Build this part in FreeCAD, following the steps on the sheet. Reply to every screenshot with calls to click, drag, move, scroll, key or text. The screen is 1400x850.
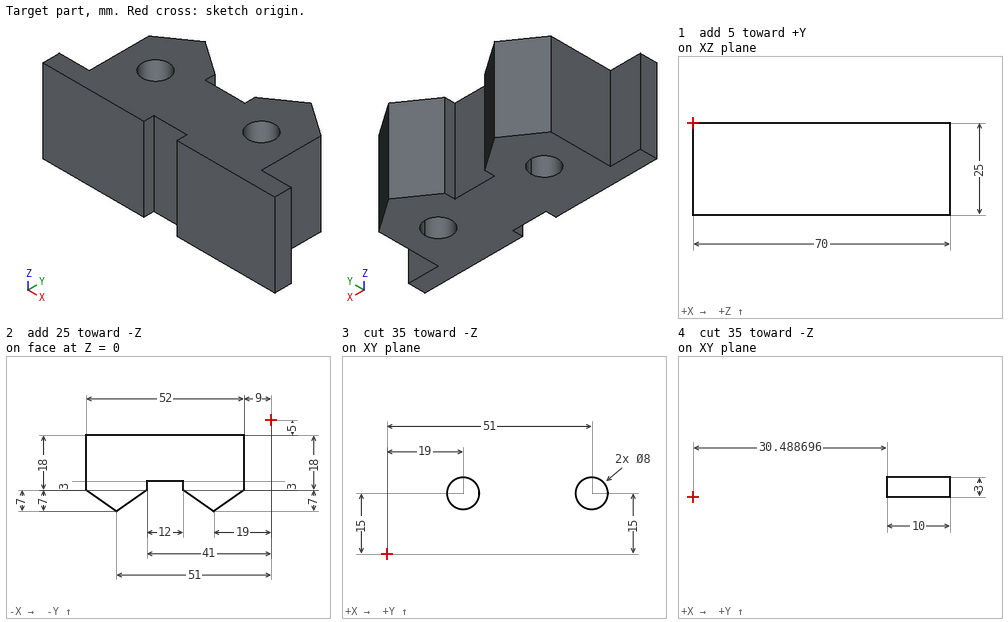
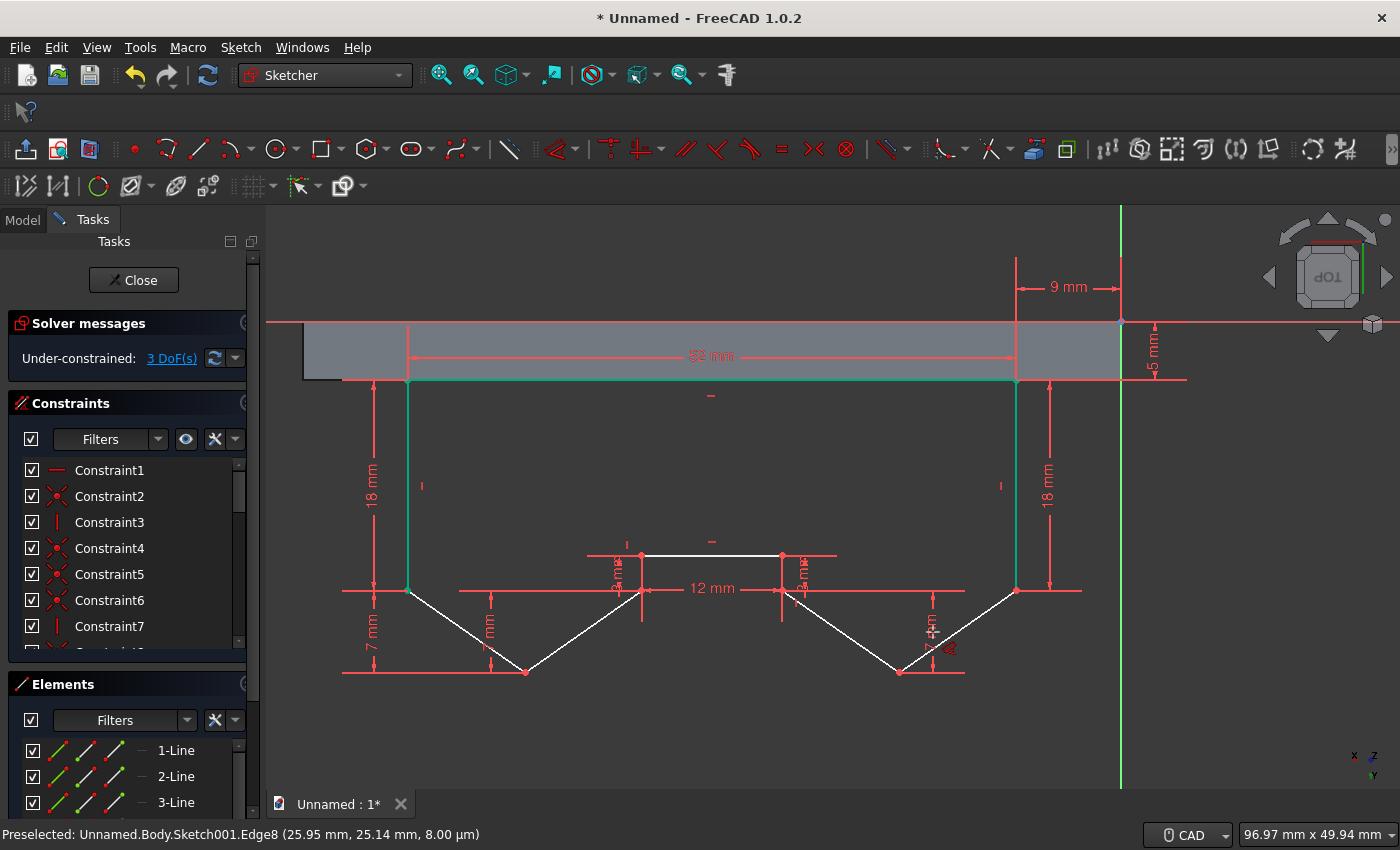
click(525, 673)
click(823, 707)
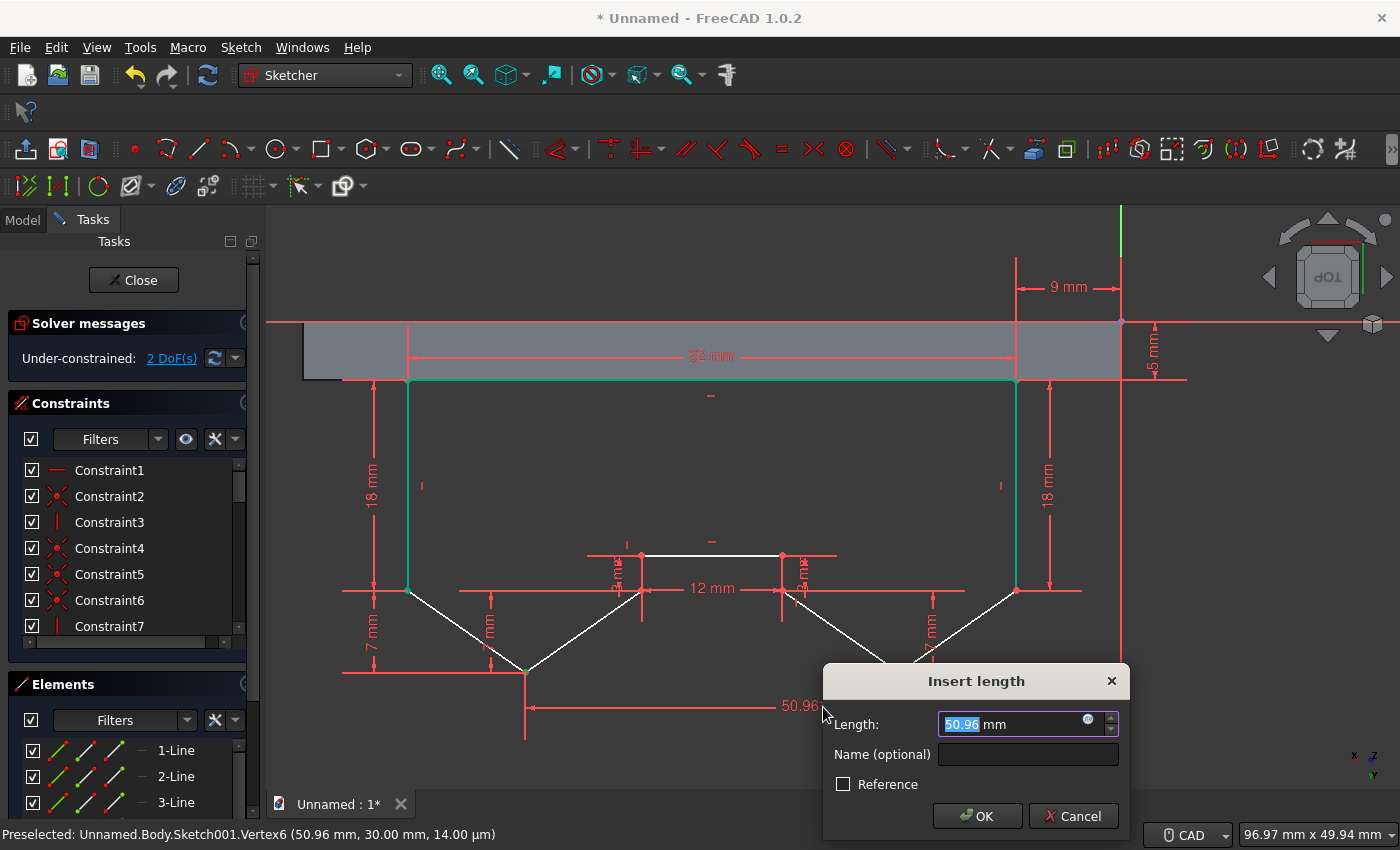
text(51)
key(Return)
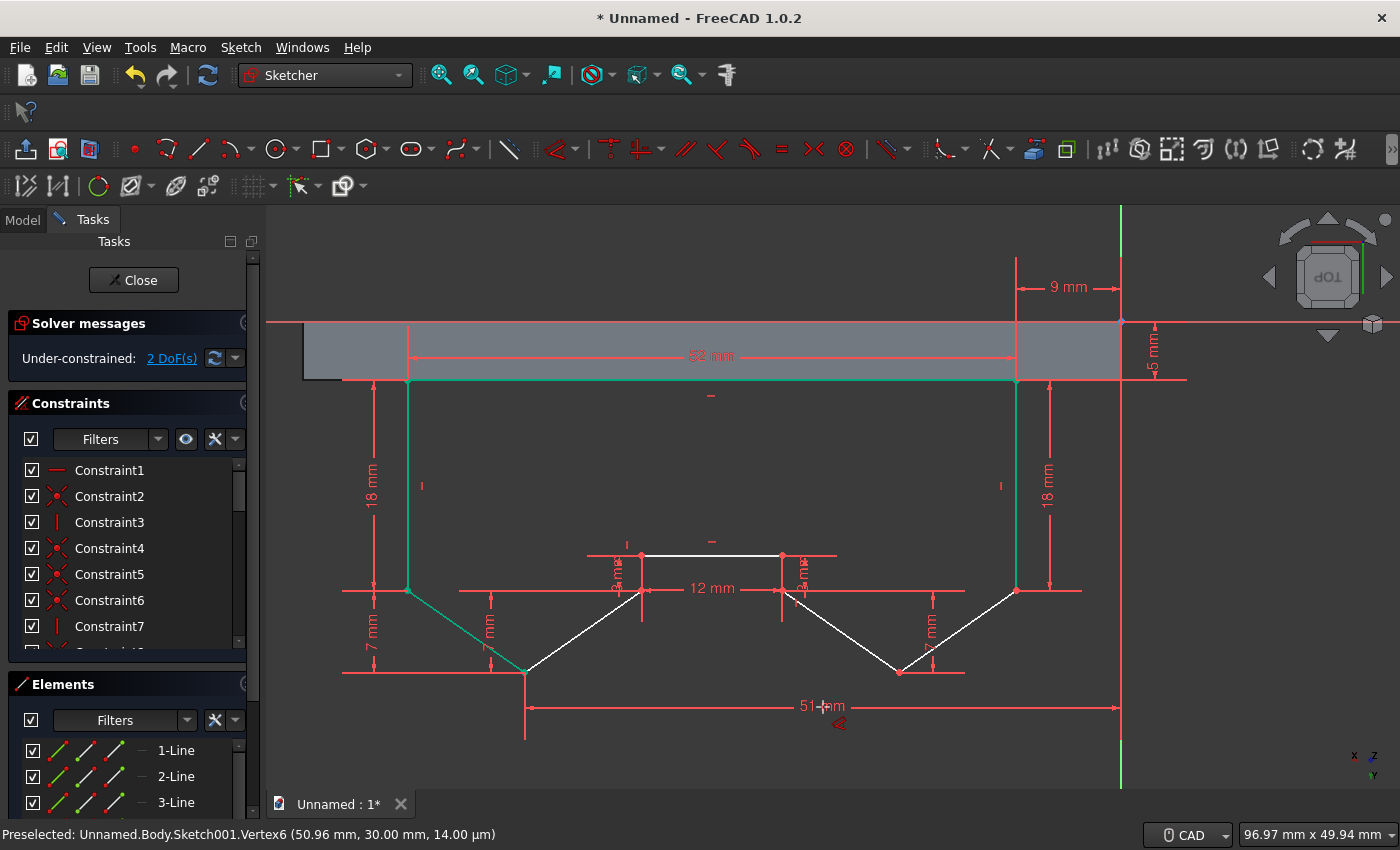
click(642, 591)
click(882, 288)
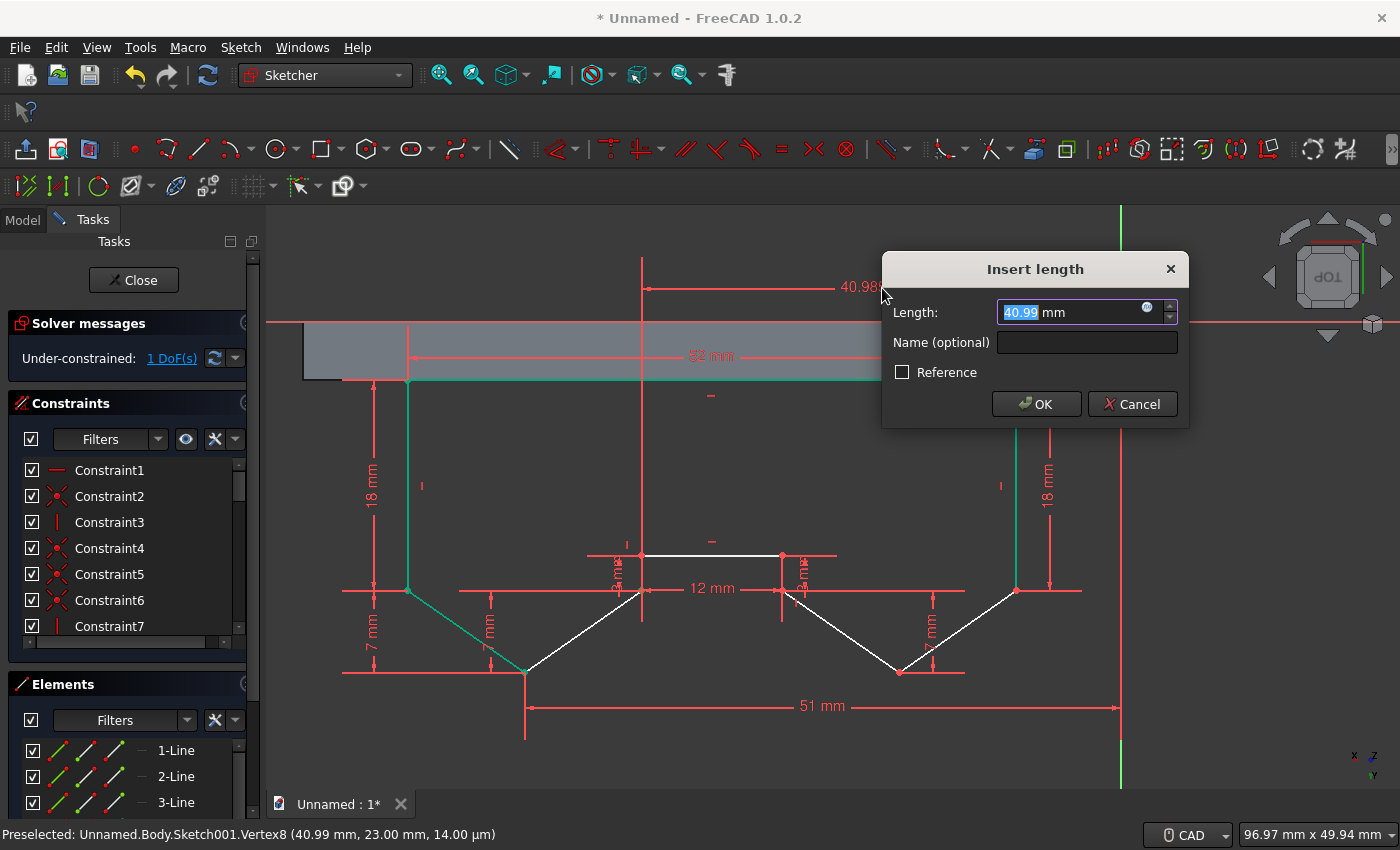
text(41)
key(Return)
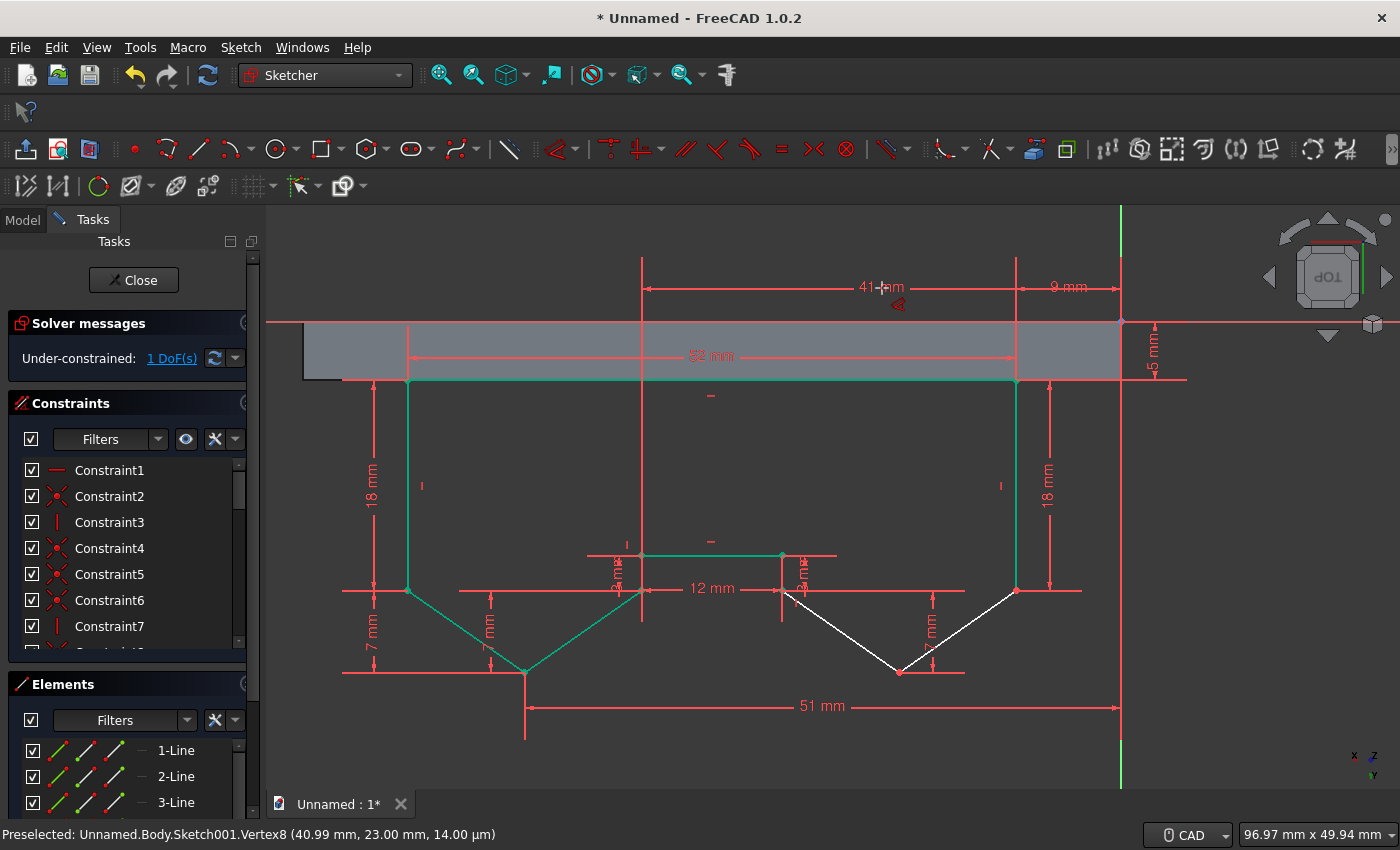
click(899, 673)
click(1010, 707)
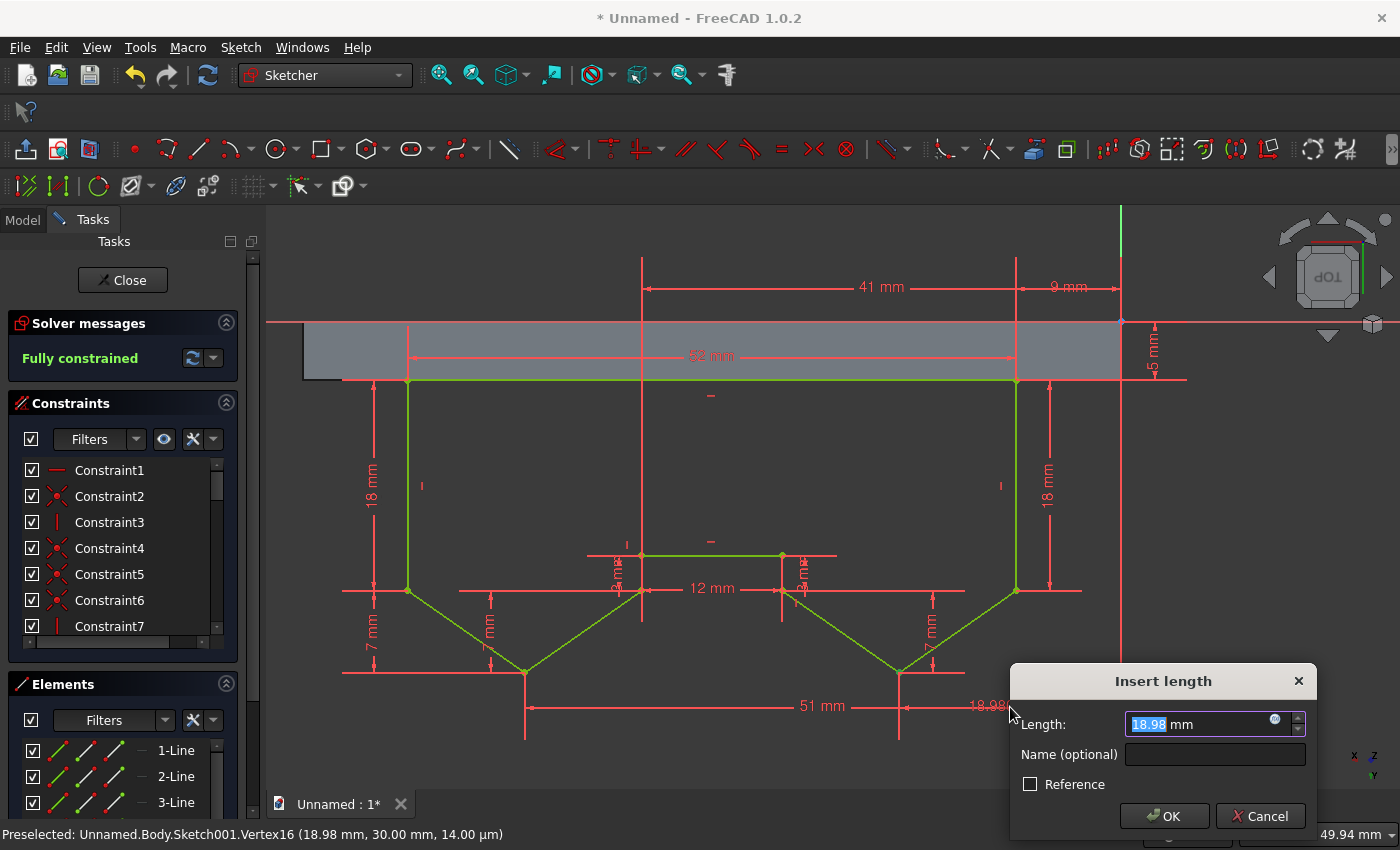
text(19)
key(Return)
key(Escape)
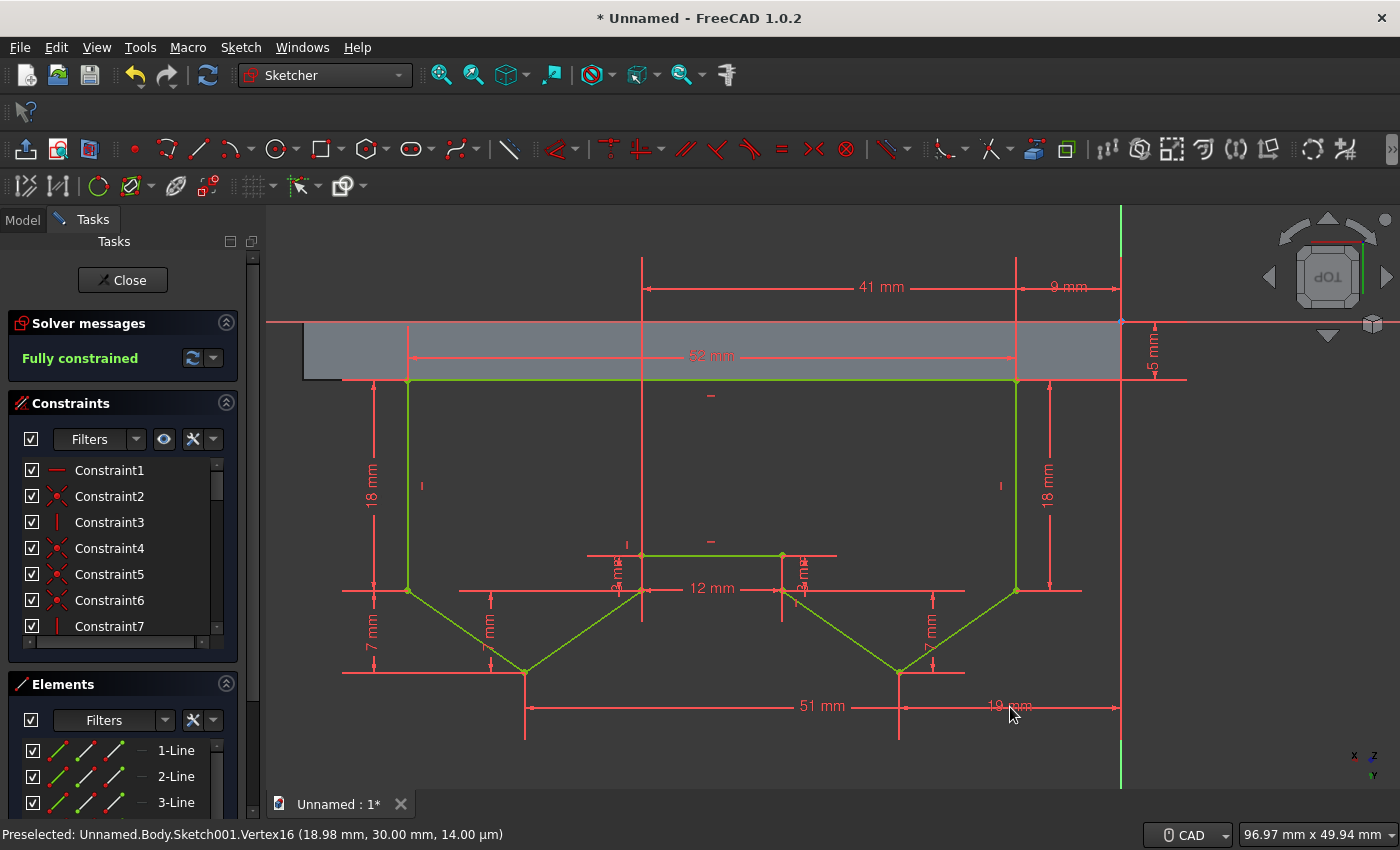
click(123, 280)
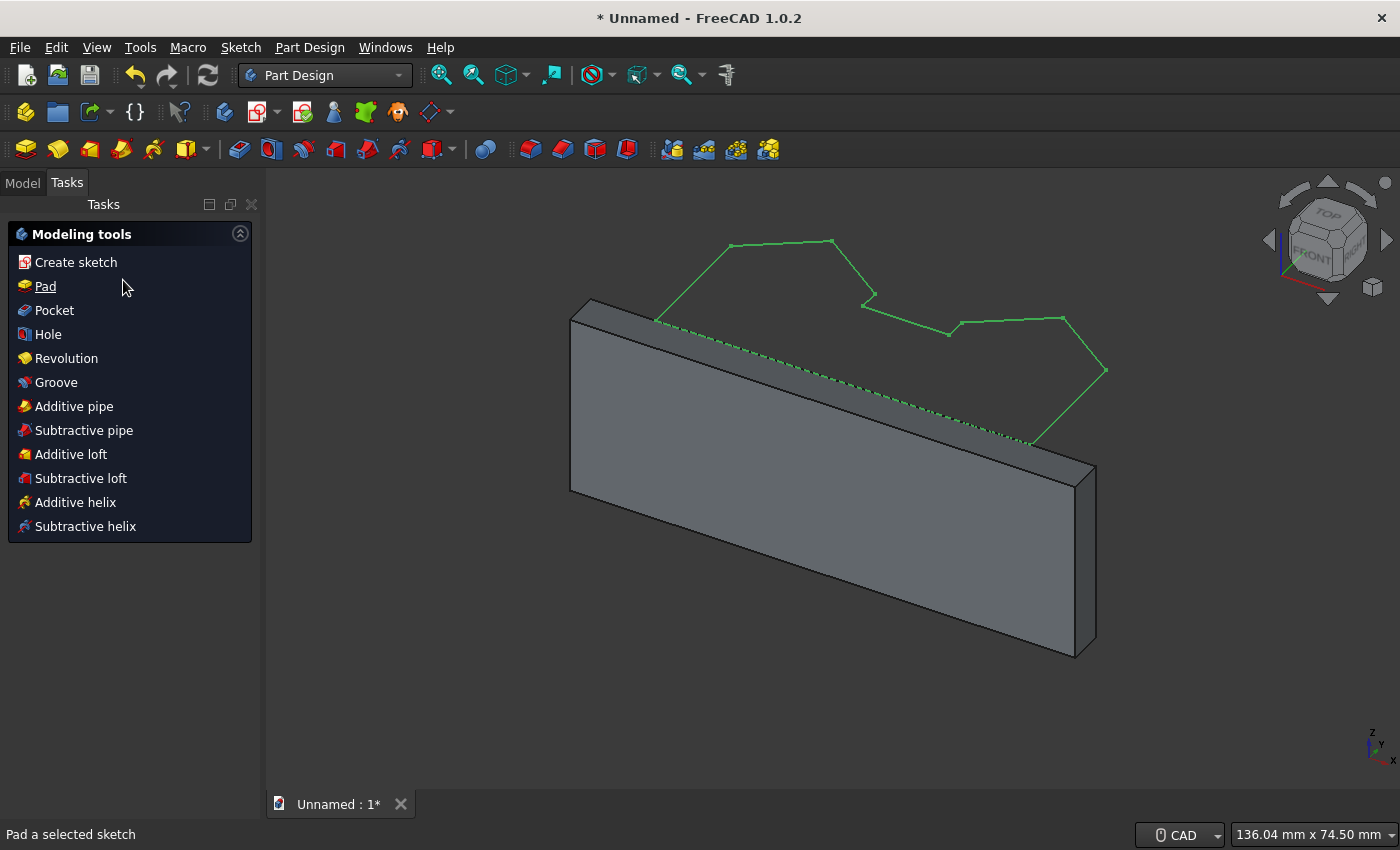
click(26, 150)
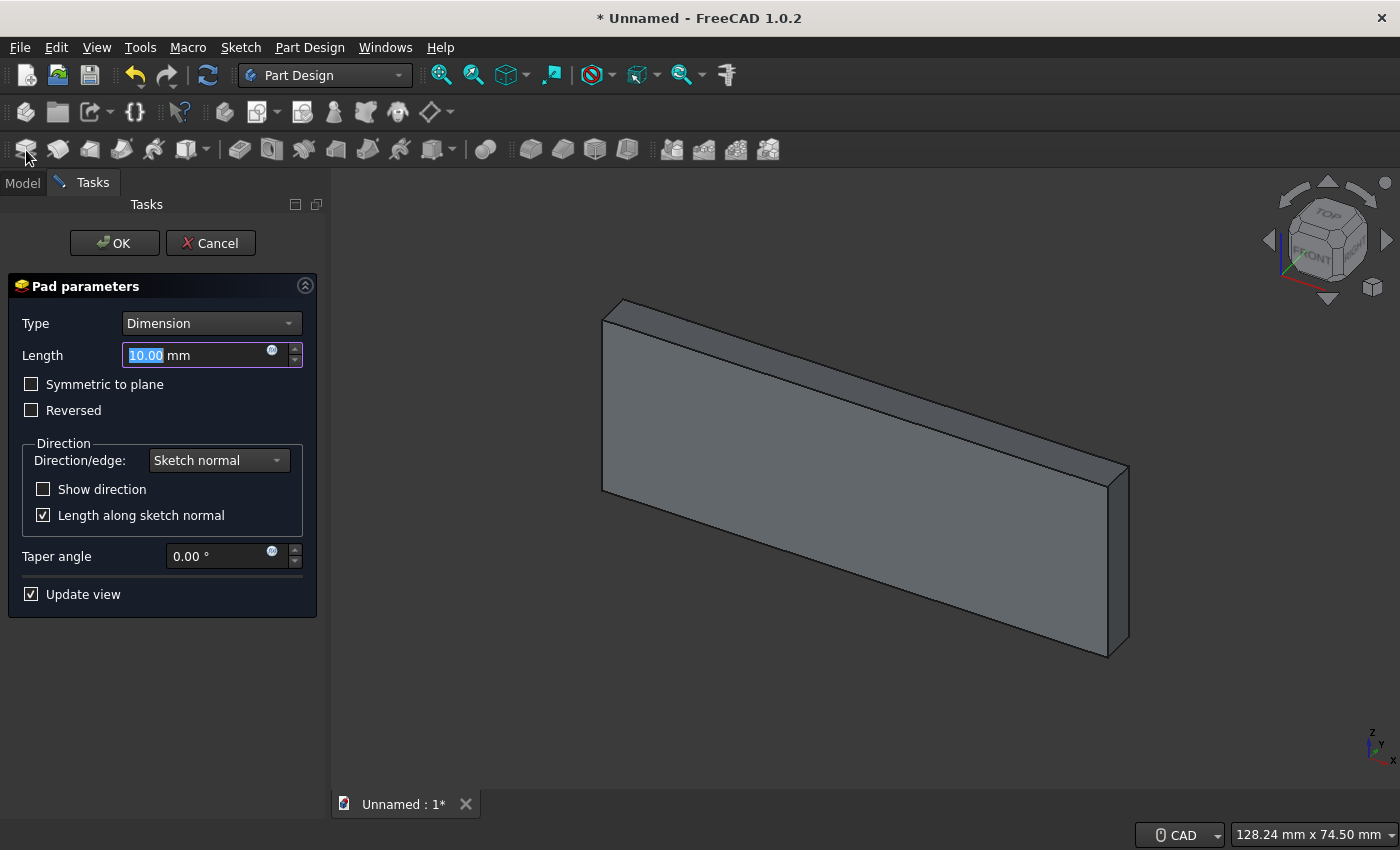
text(25)
key(Tab)